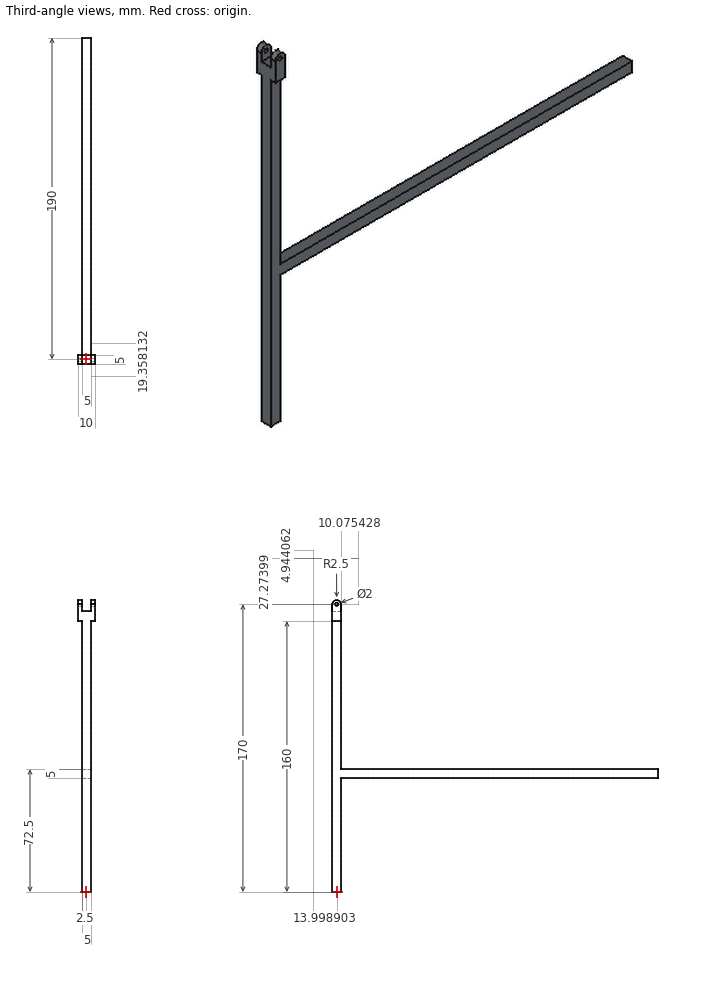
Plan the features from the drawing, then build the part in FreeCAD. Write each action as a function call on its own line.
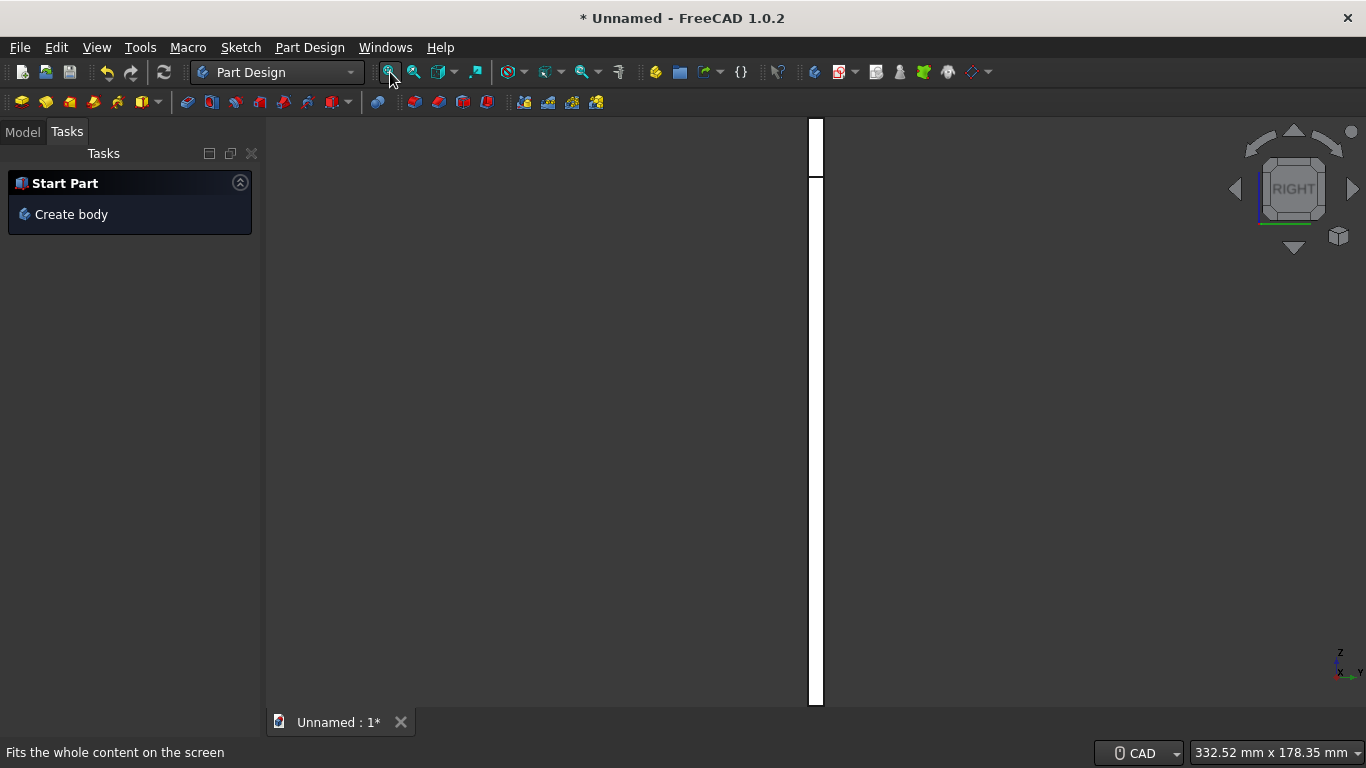
click(816, 146)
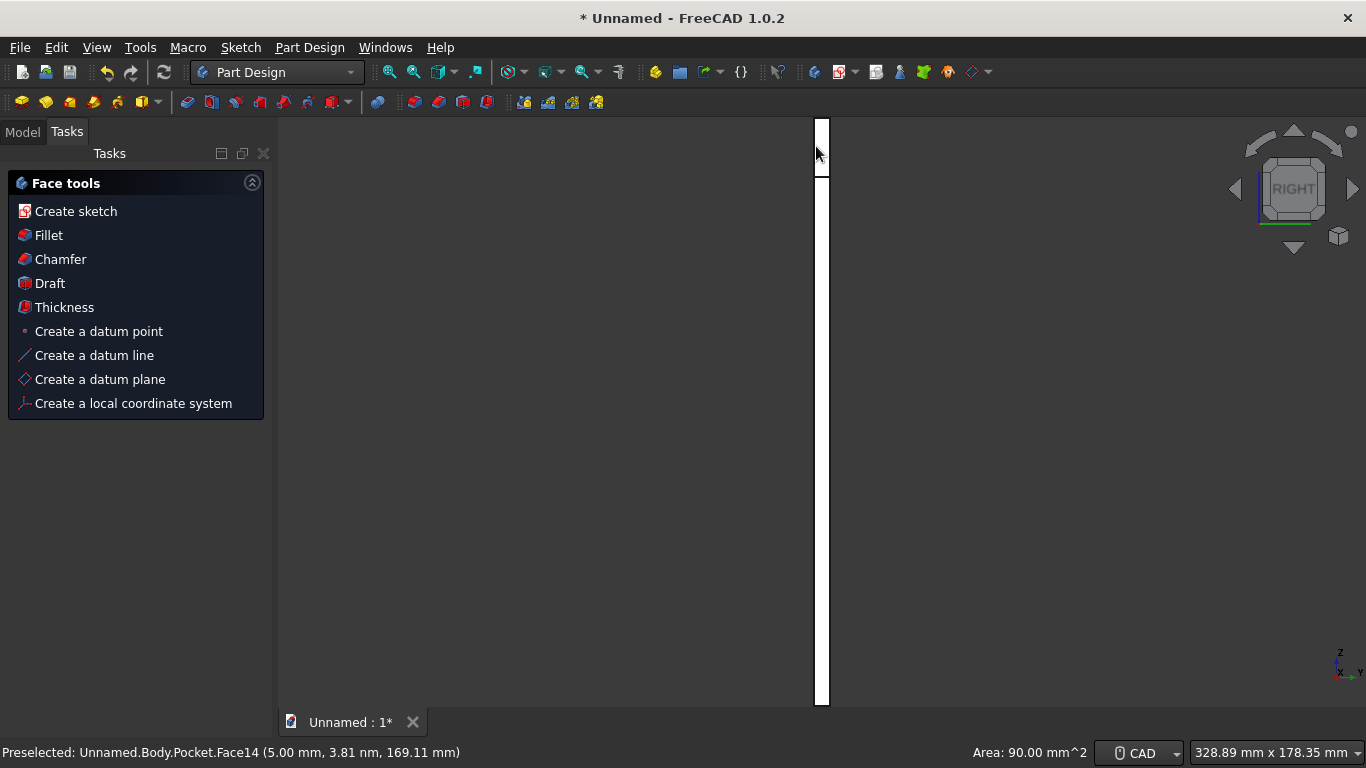
click(840, 72)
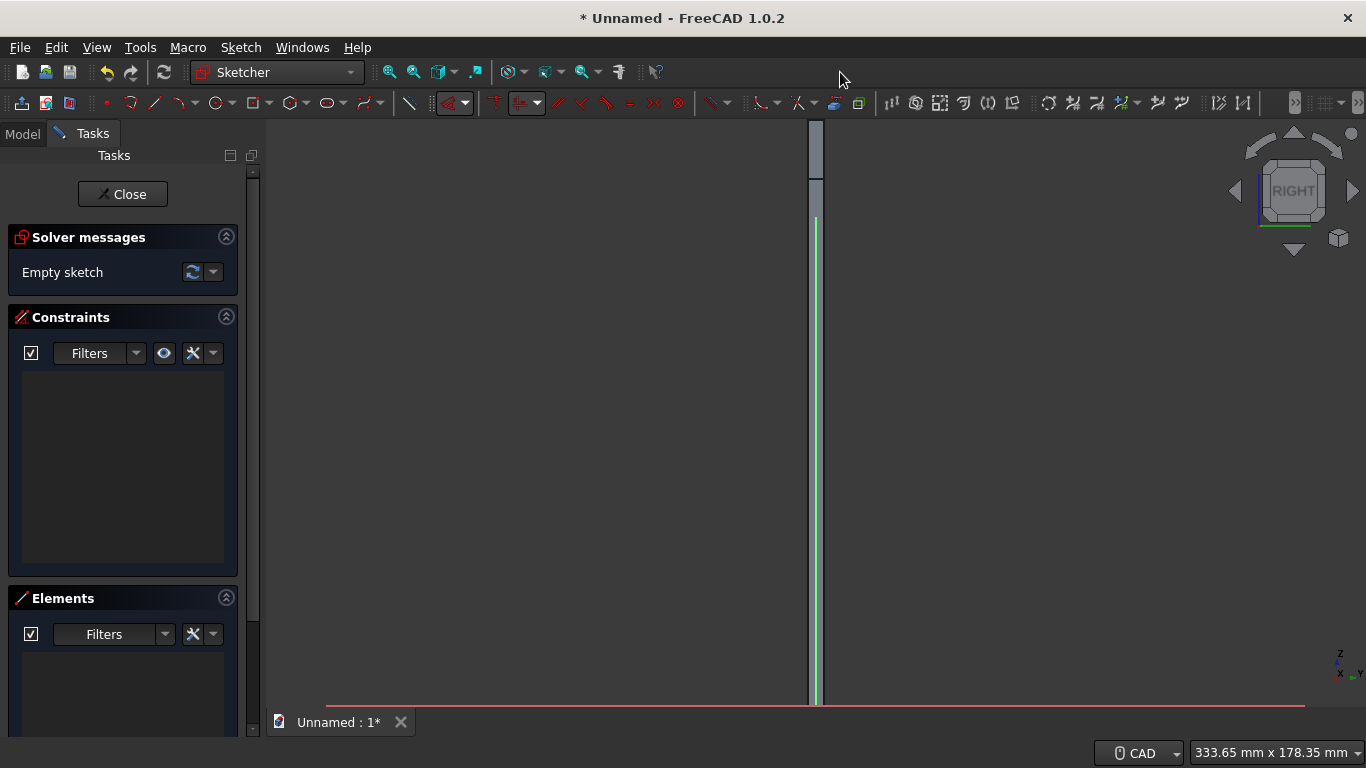
scroll(748, 413, down, 5)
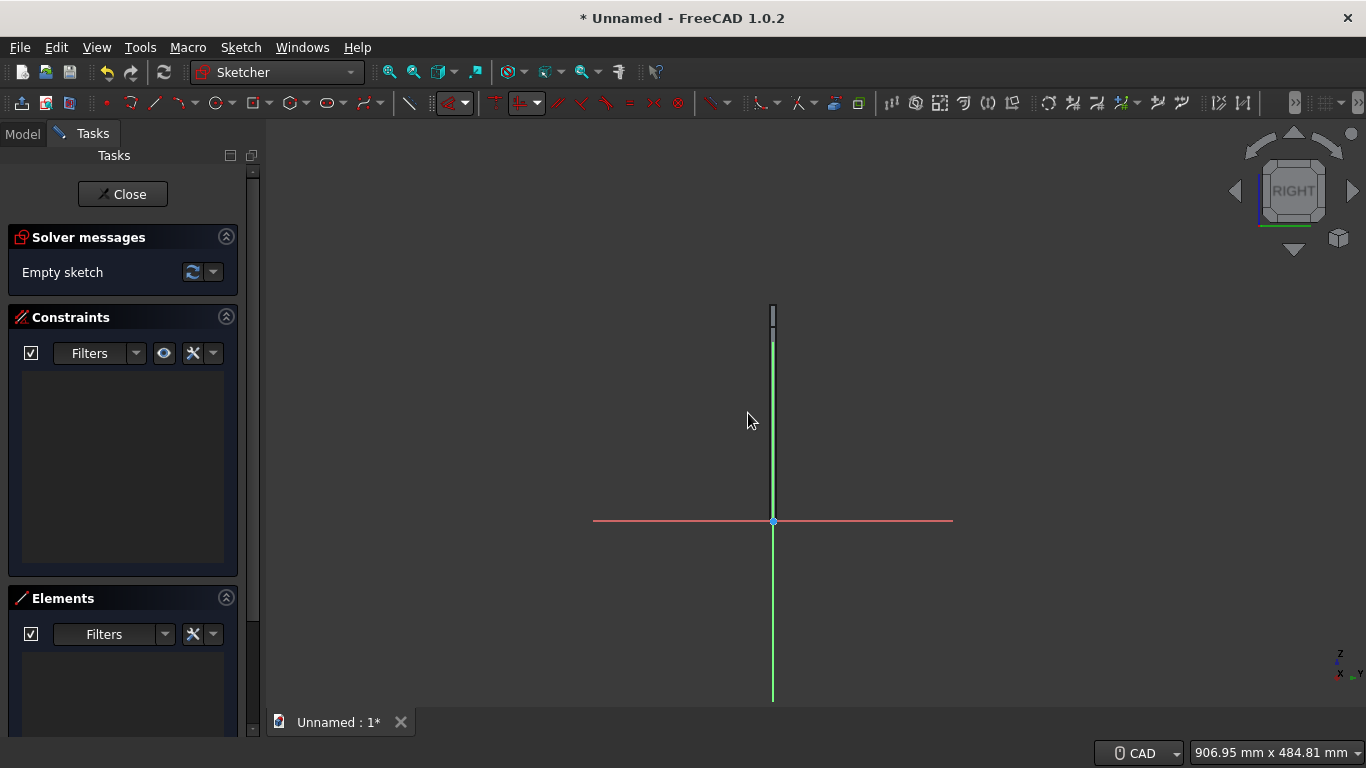
scroll(776, 282, up, 11)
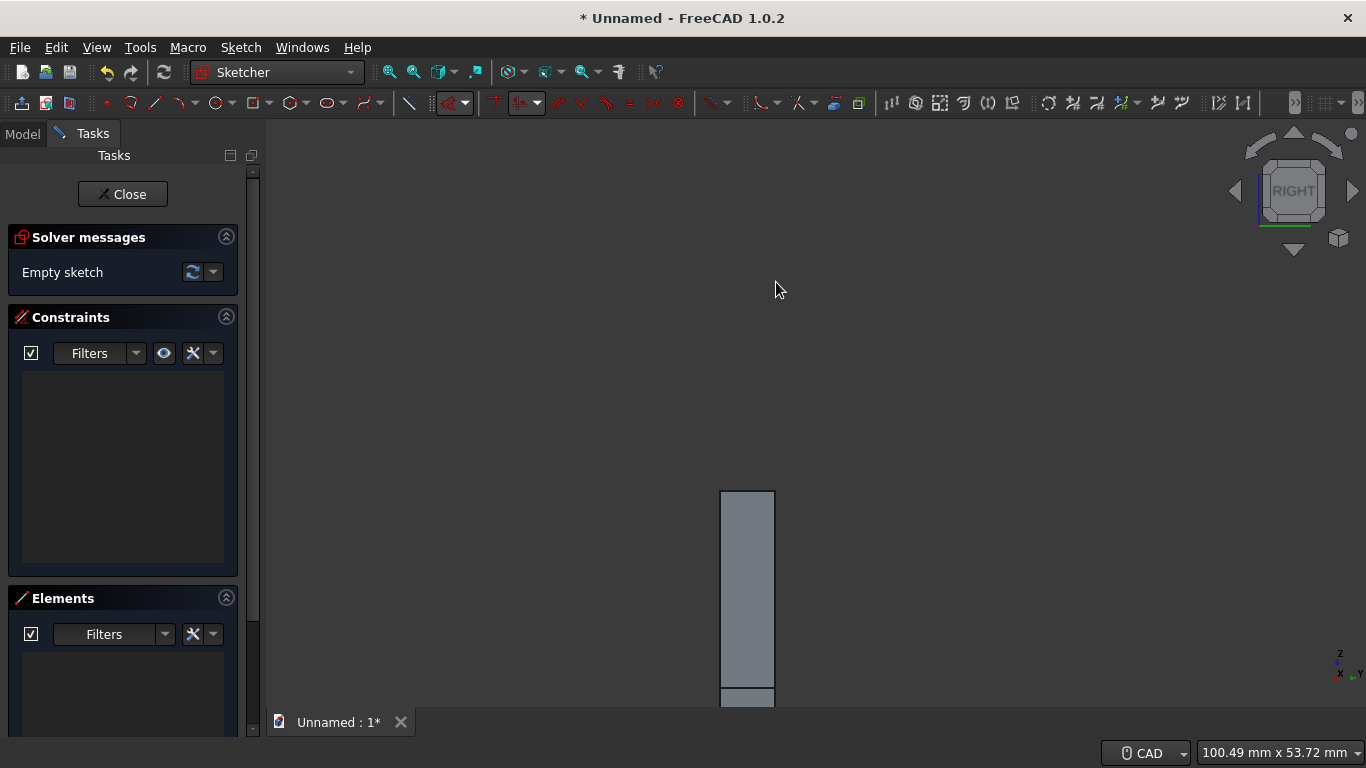
click(132, 104)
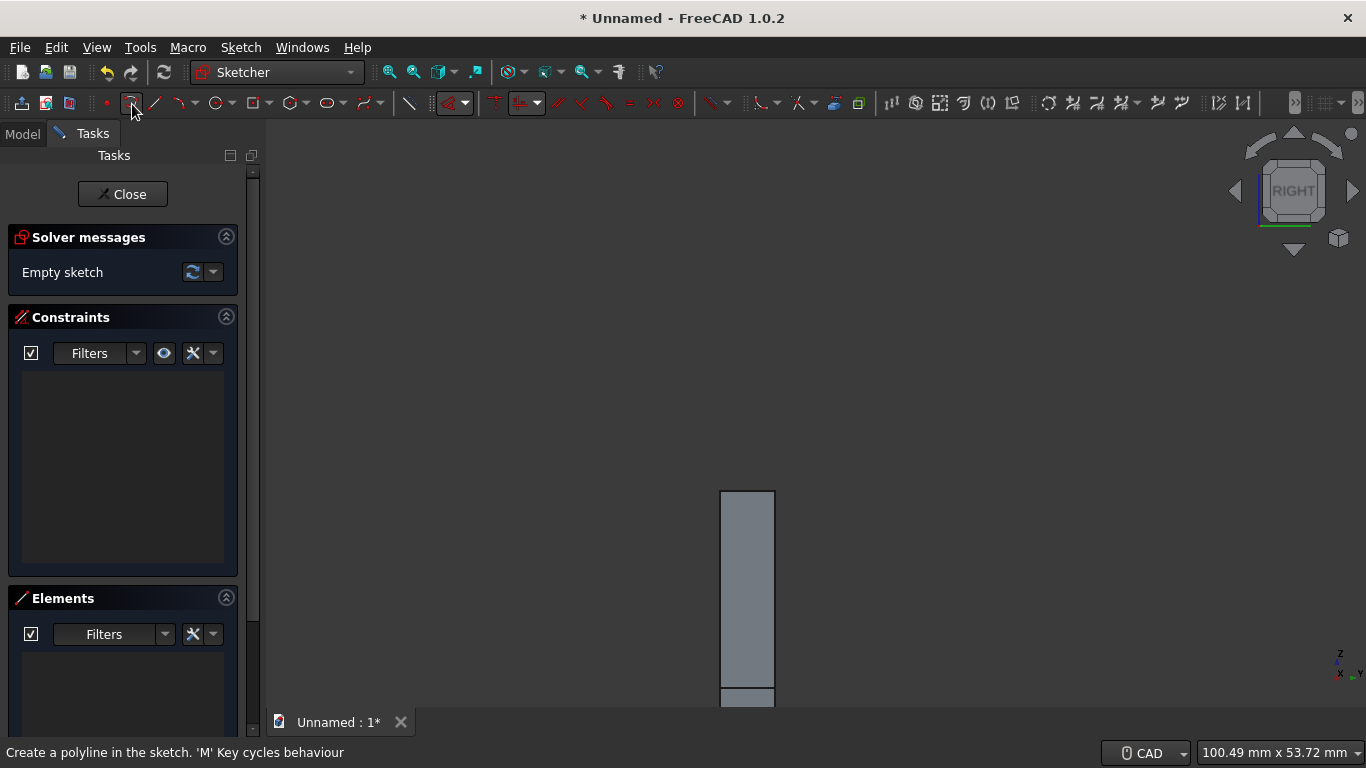
click(775, 578)
click(885, 578)
click(885, 280)
click(595, 226)
click(720, 578)
right_click(720, 578)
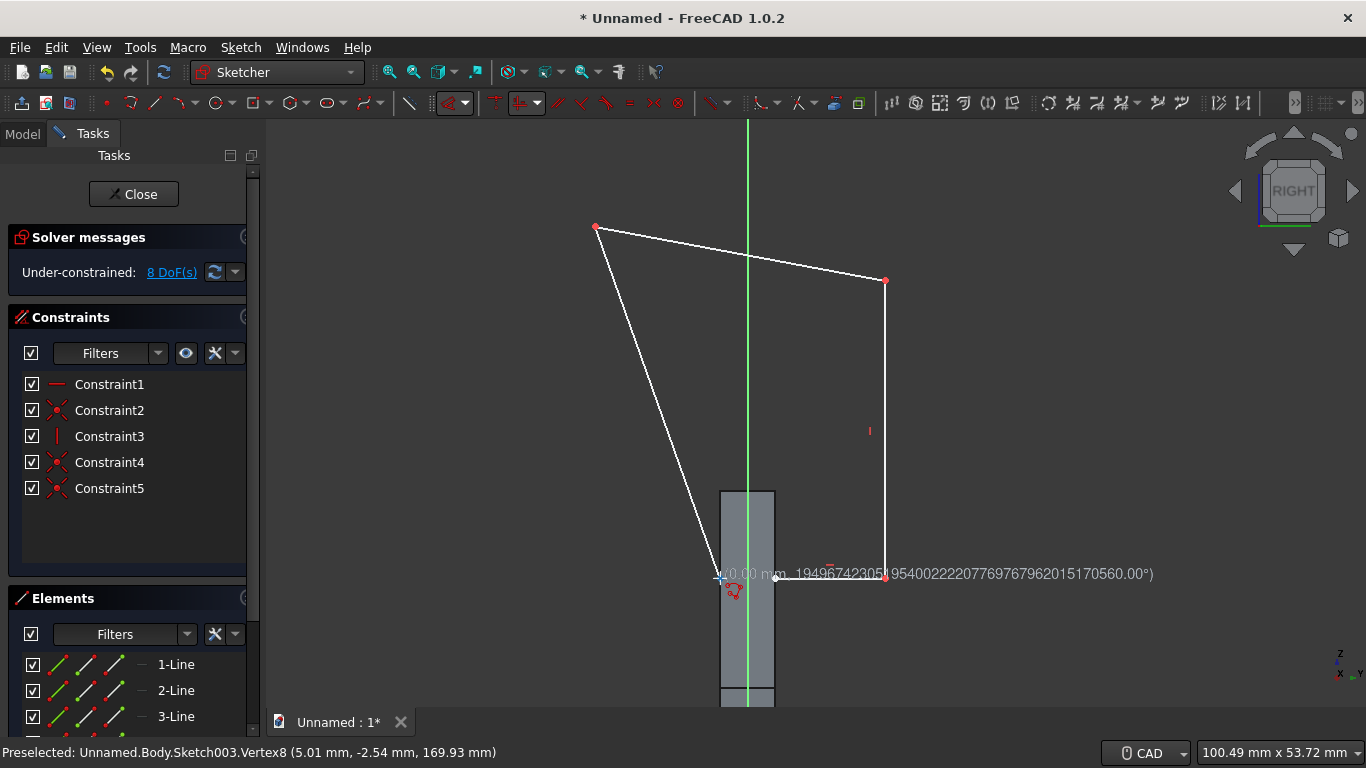
click(180, 104)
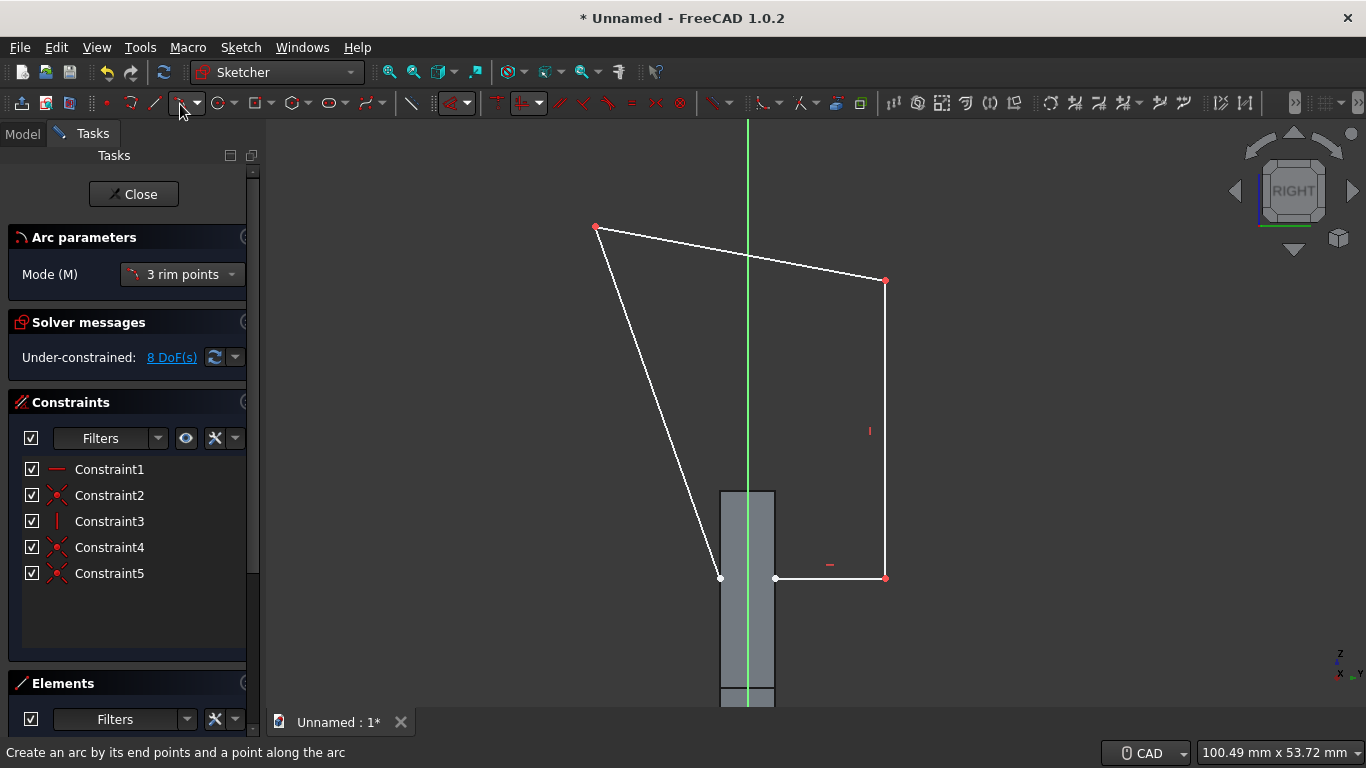
click(720, 579)
click(775, 579)
click(764, 556)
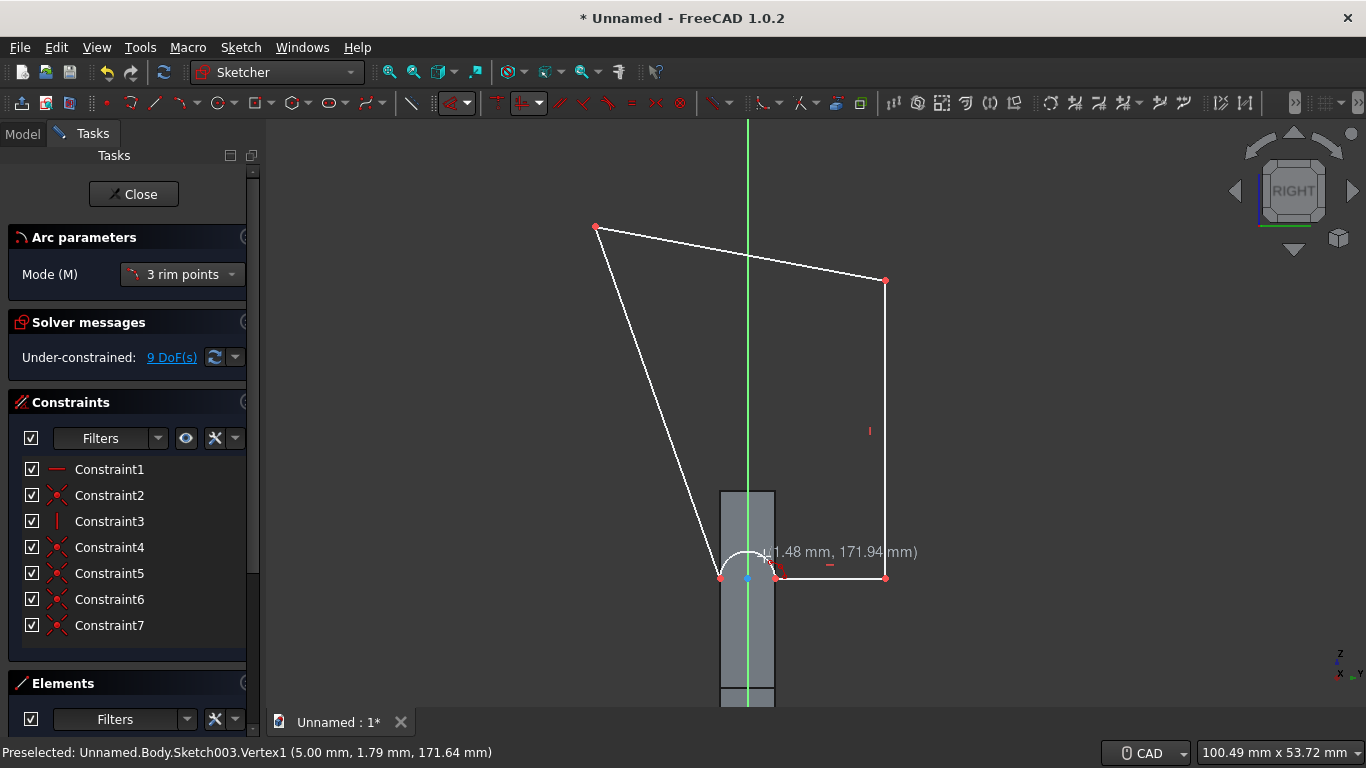
click(218, 104)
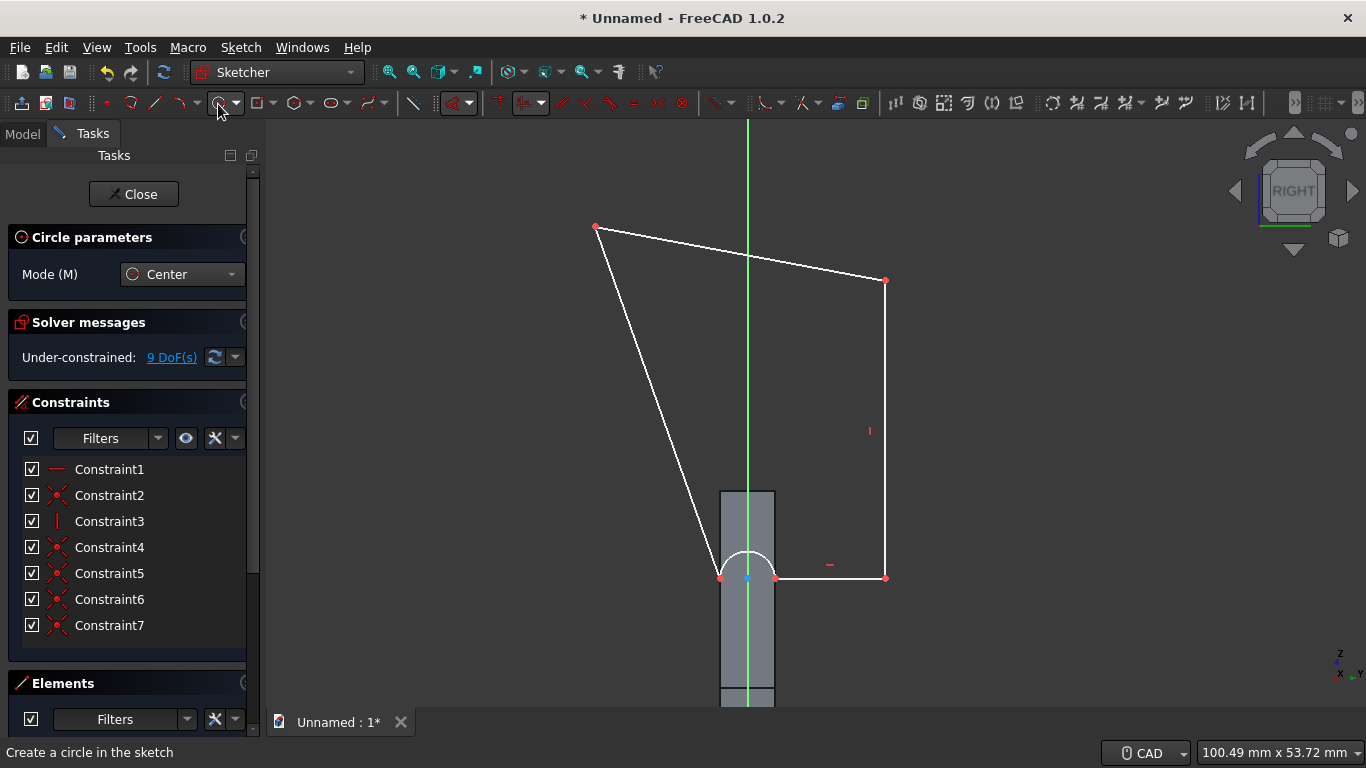
scroll(748, 578, up, 4)